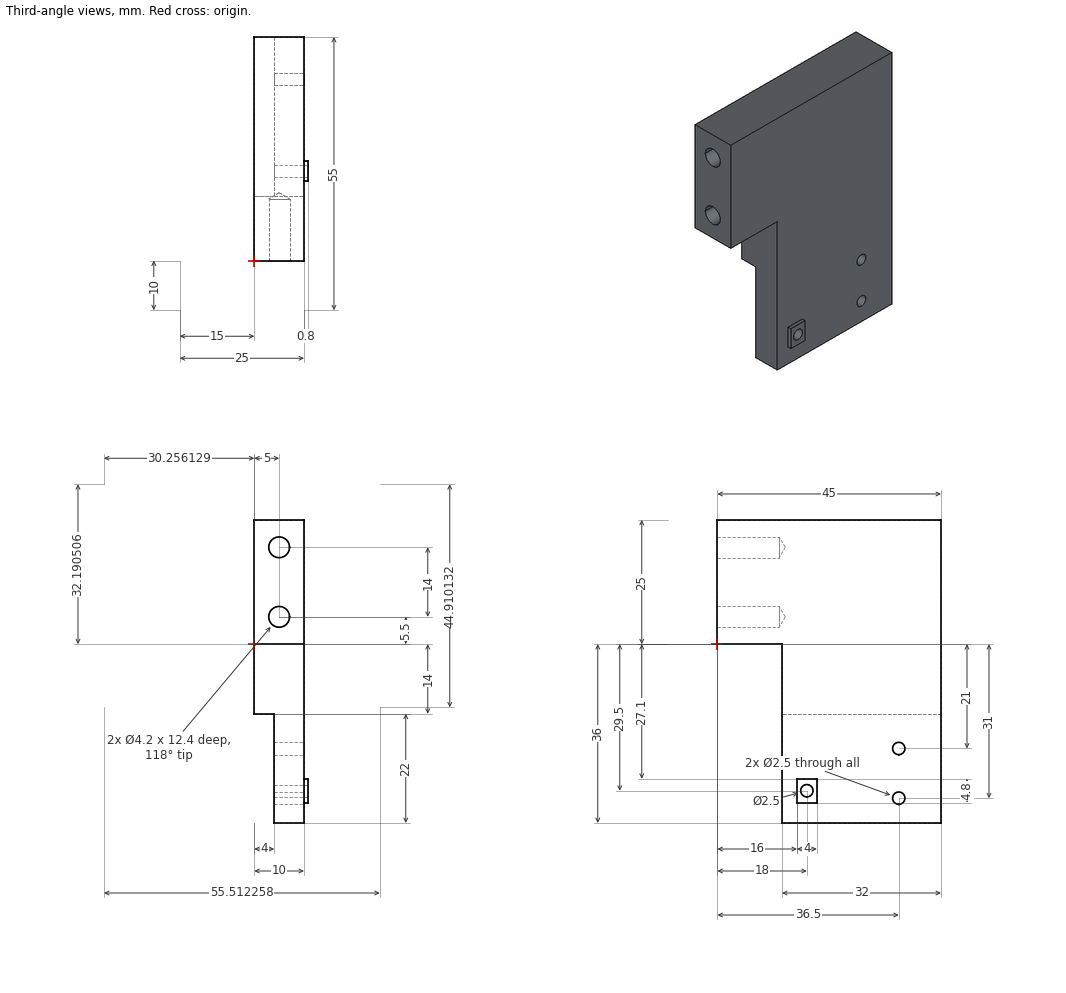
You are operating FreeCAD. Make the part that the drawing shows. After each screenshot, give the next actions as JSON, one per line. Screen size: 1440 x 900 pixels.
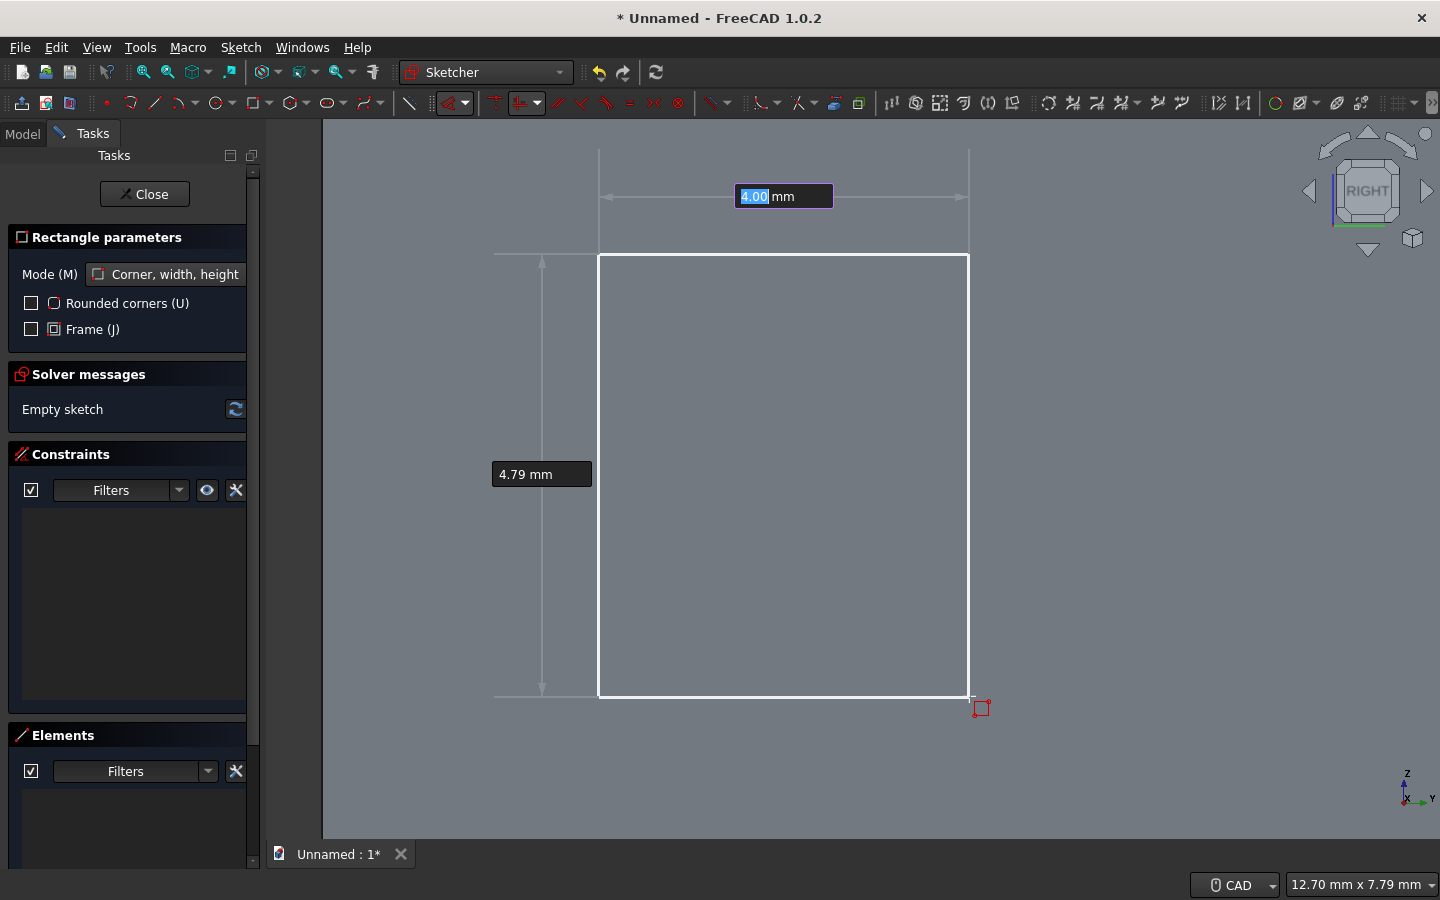
{"action": "type", "text": "4"}
{"action": "key", "text": "Tab"}
{"action": "type", "text": "4.8"}
{"action": "key", "text": "Return"}
{"action": "key", "text": "Escape"}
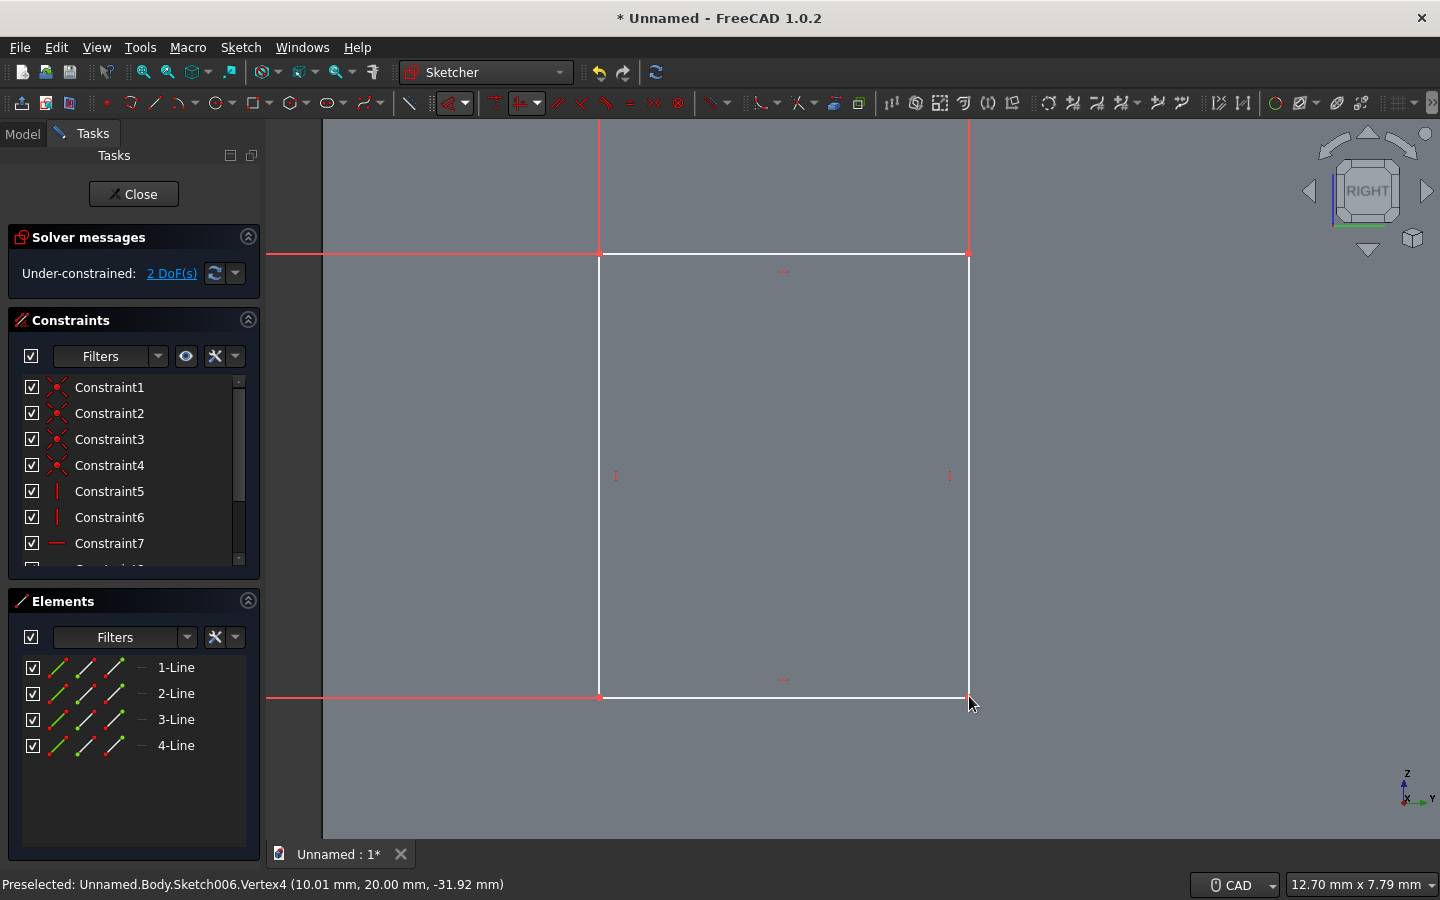
{"action": "left_click", "coordinate": [599, 254]}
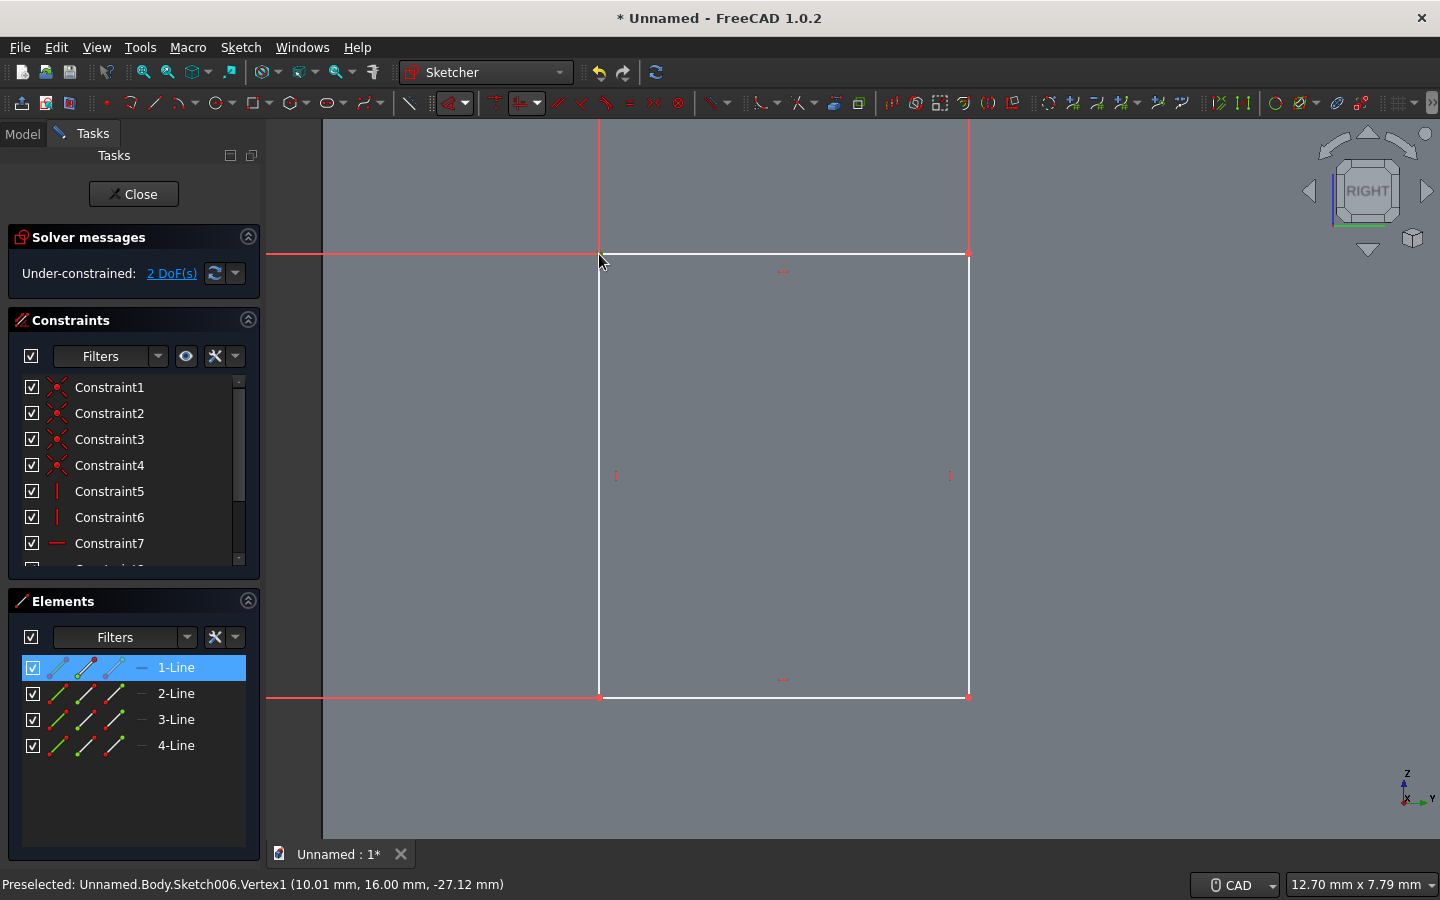
{"action": "key", "text": "l"}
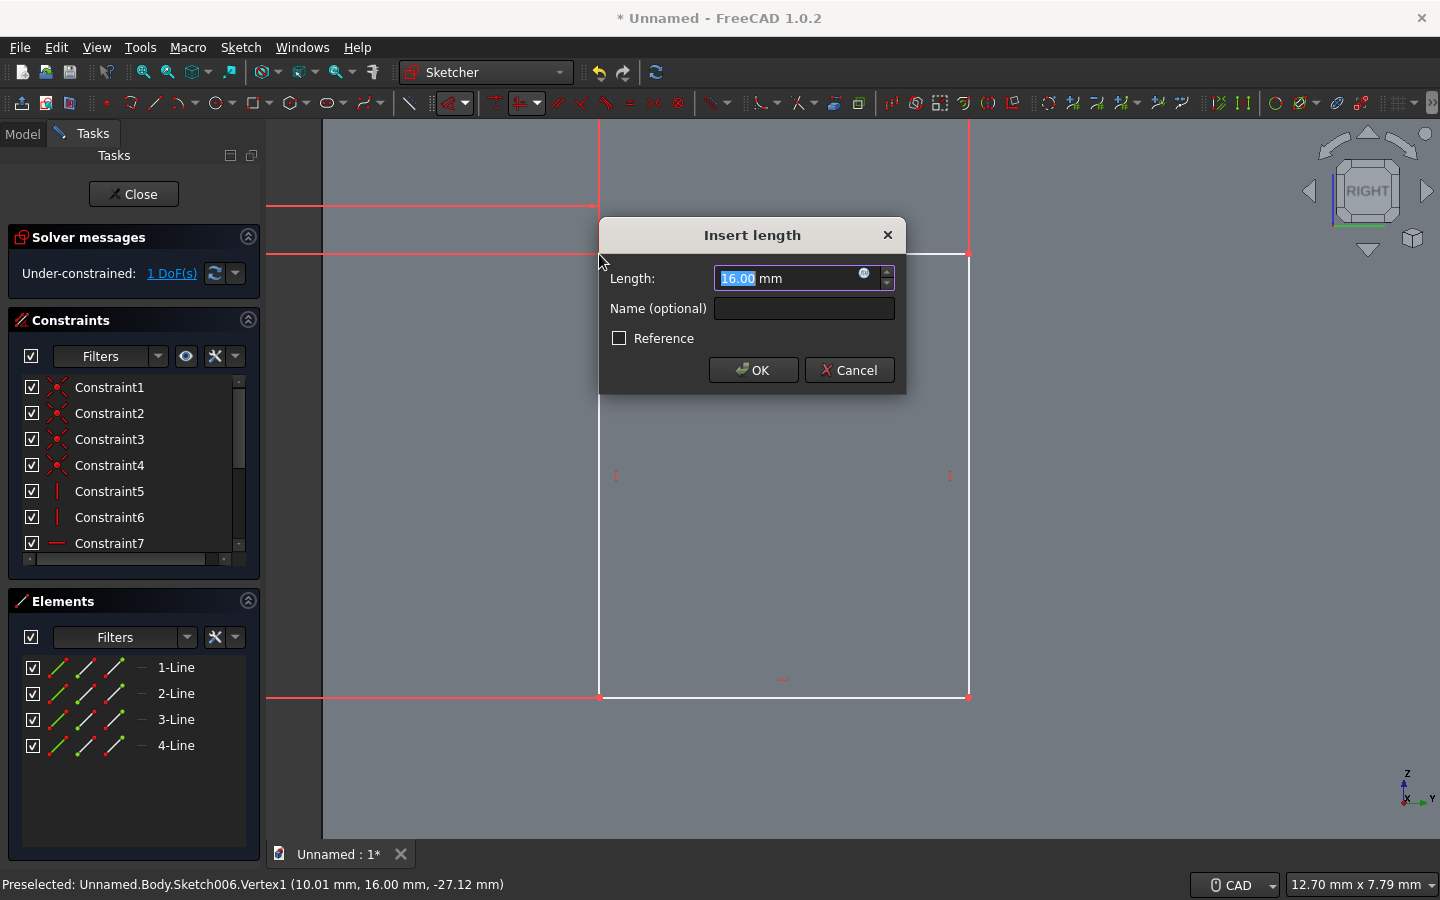
{"action": "type", "text": "16"}
{"action": "key", "text": "Return"}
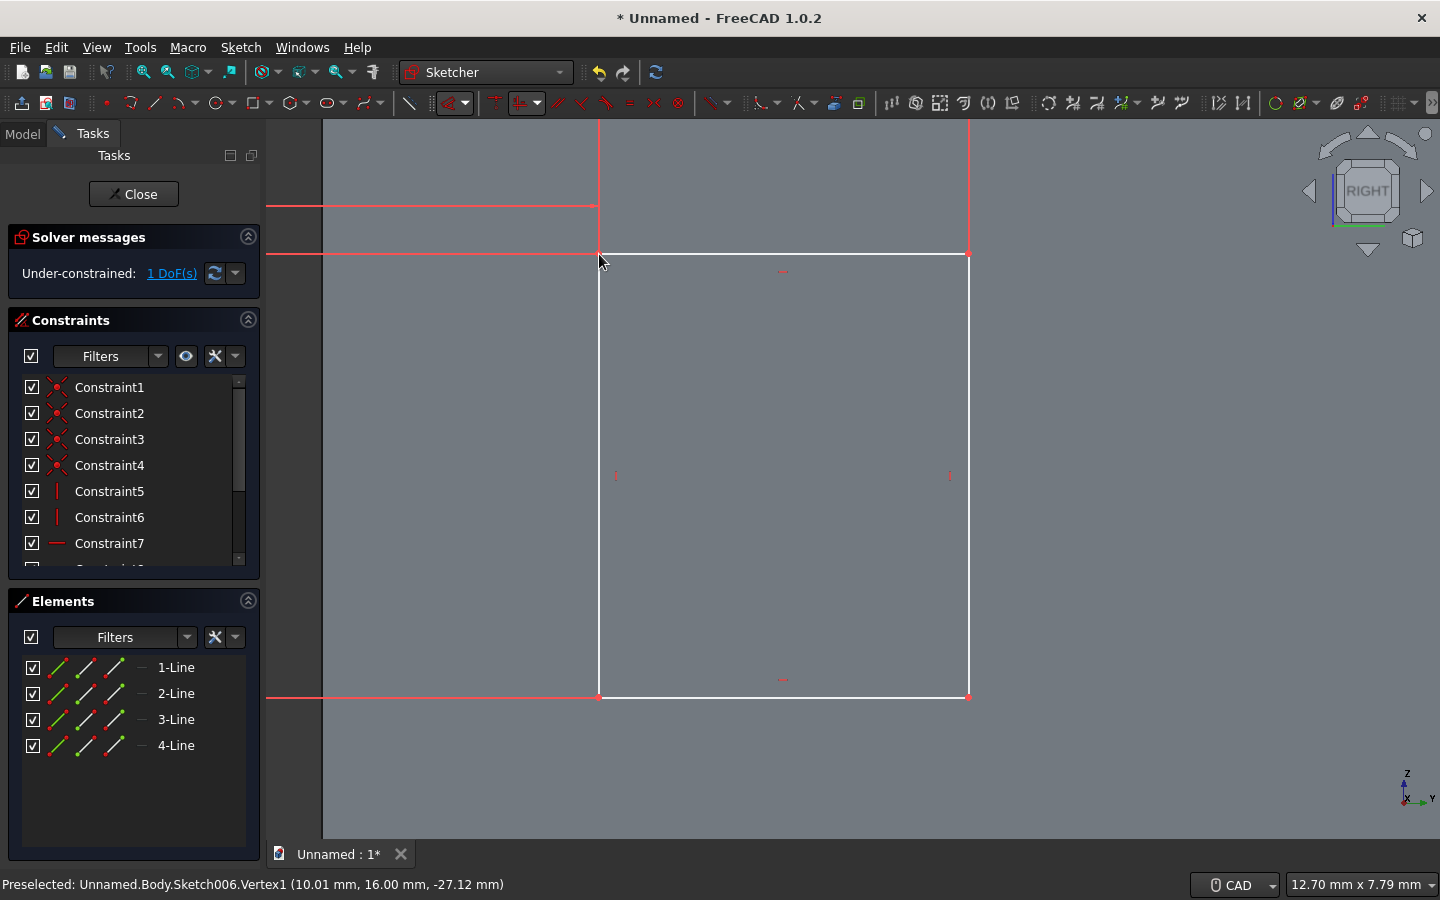
{"action": "left_click", "coordinate": [599, 254]}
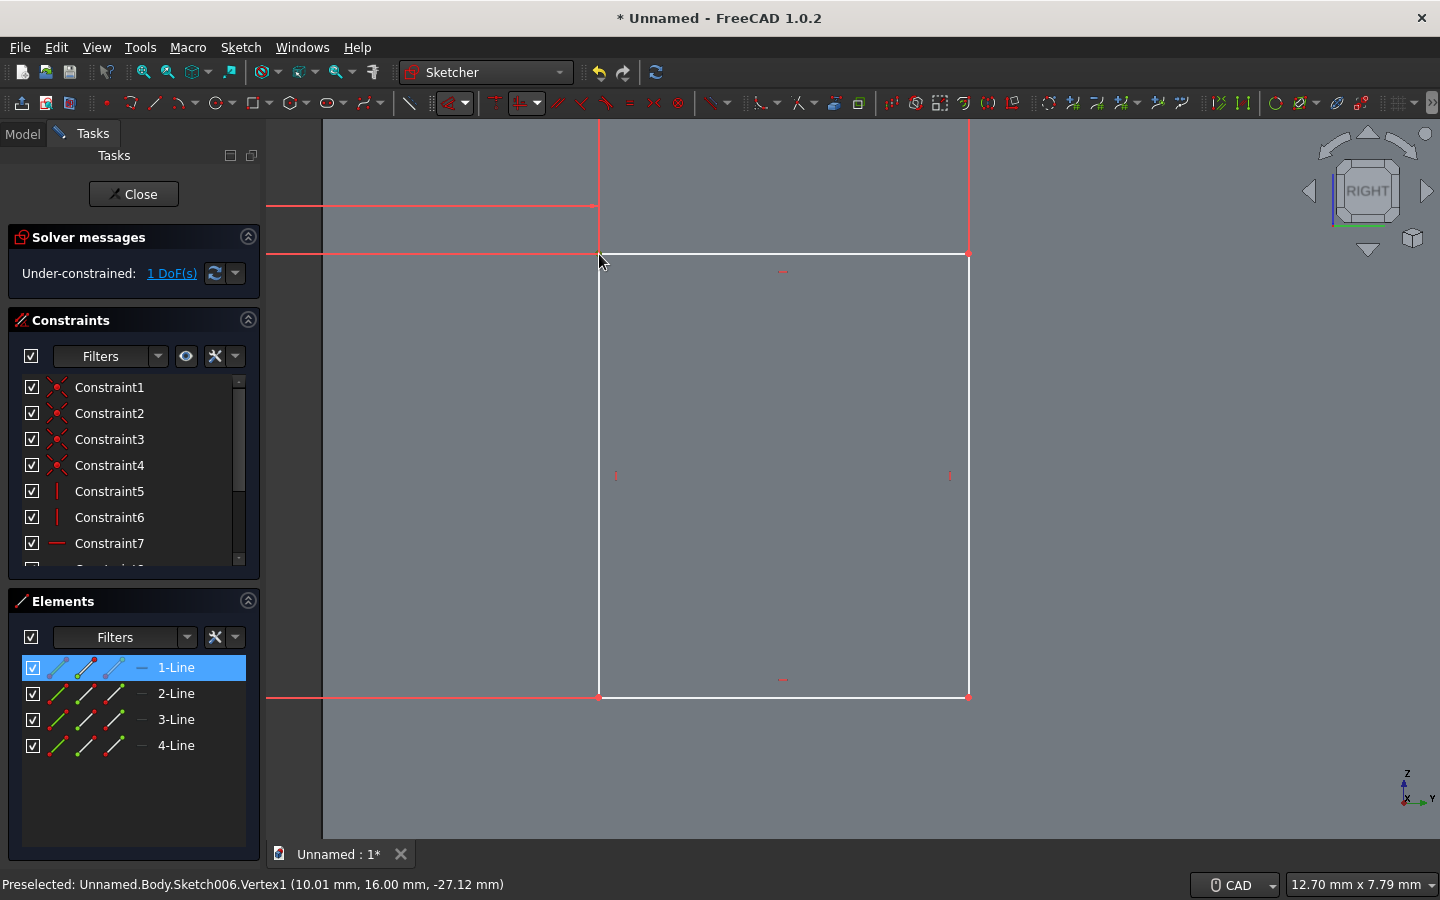
{"action": "key", "text": "i"}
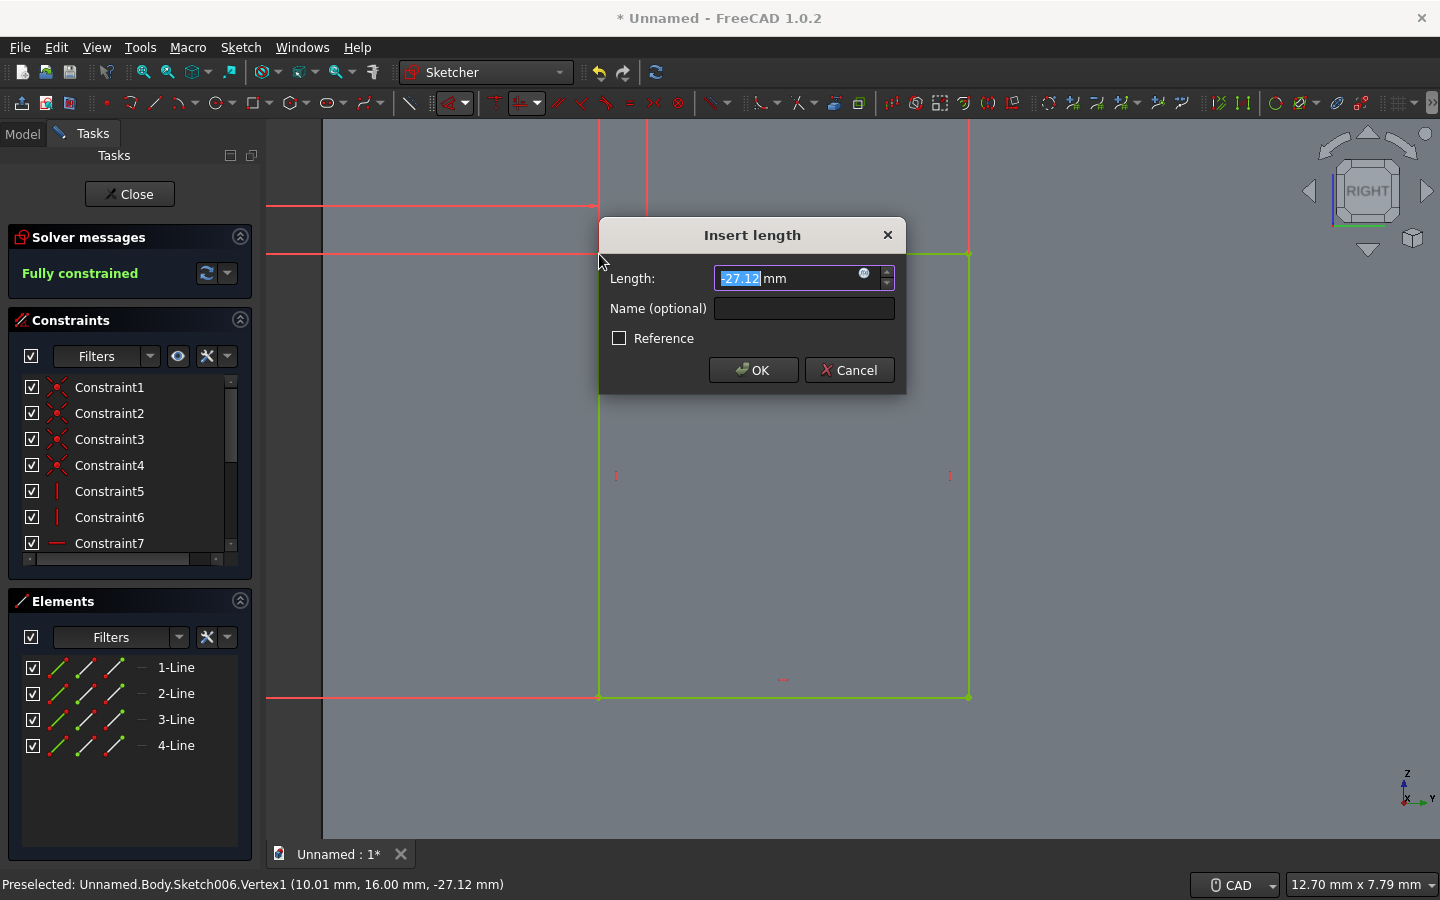
{"action": "type", "text": "-27.1"}
{"action": "key", "text": "Return"}